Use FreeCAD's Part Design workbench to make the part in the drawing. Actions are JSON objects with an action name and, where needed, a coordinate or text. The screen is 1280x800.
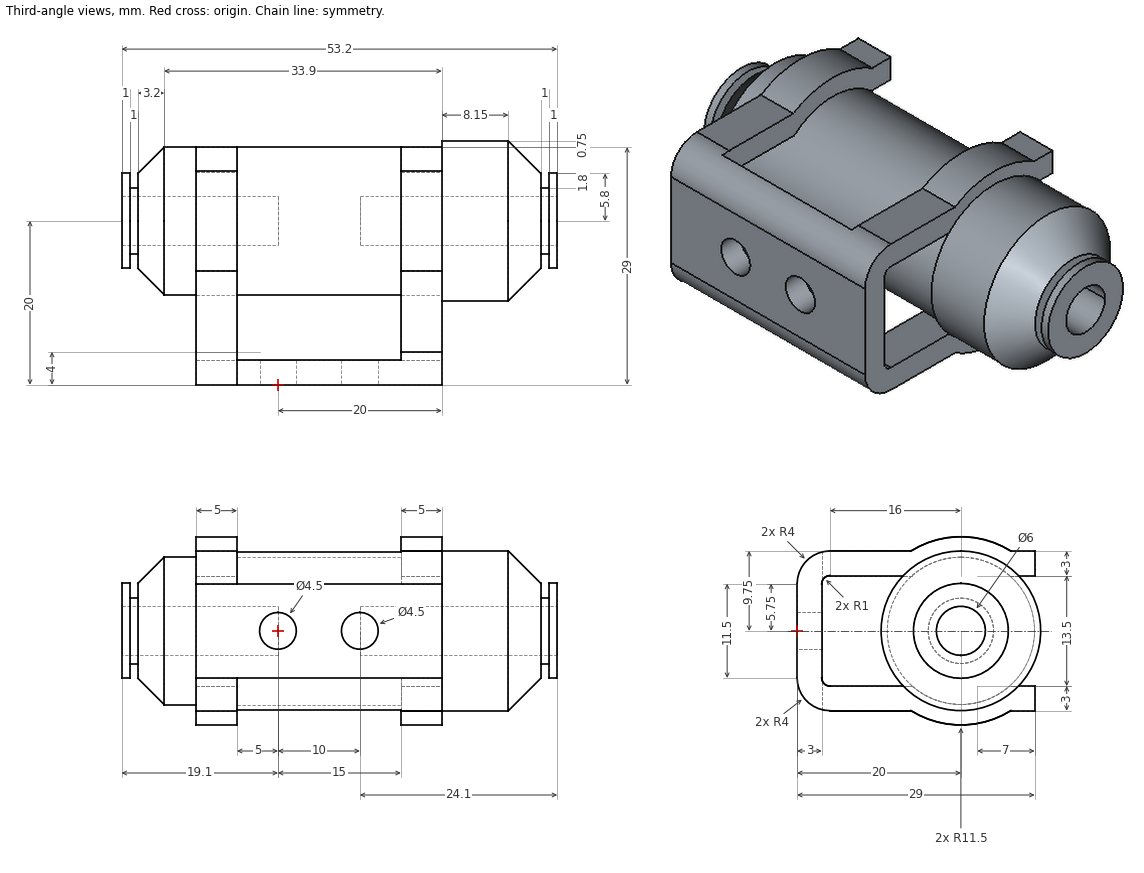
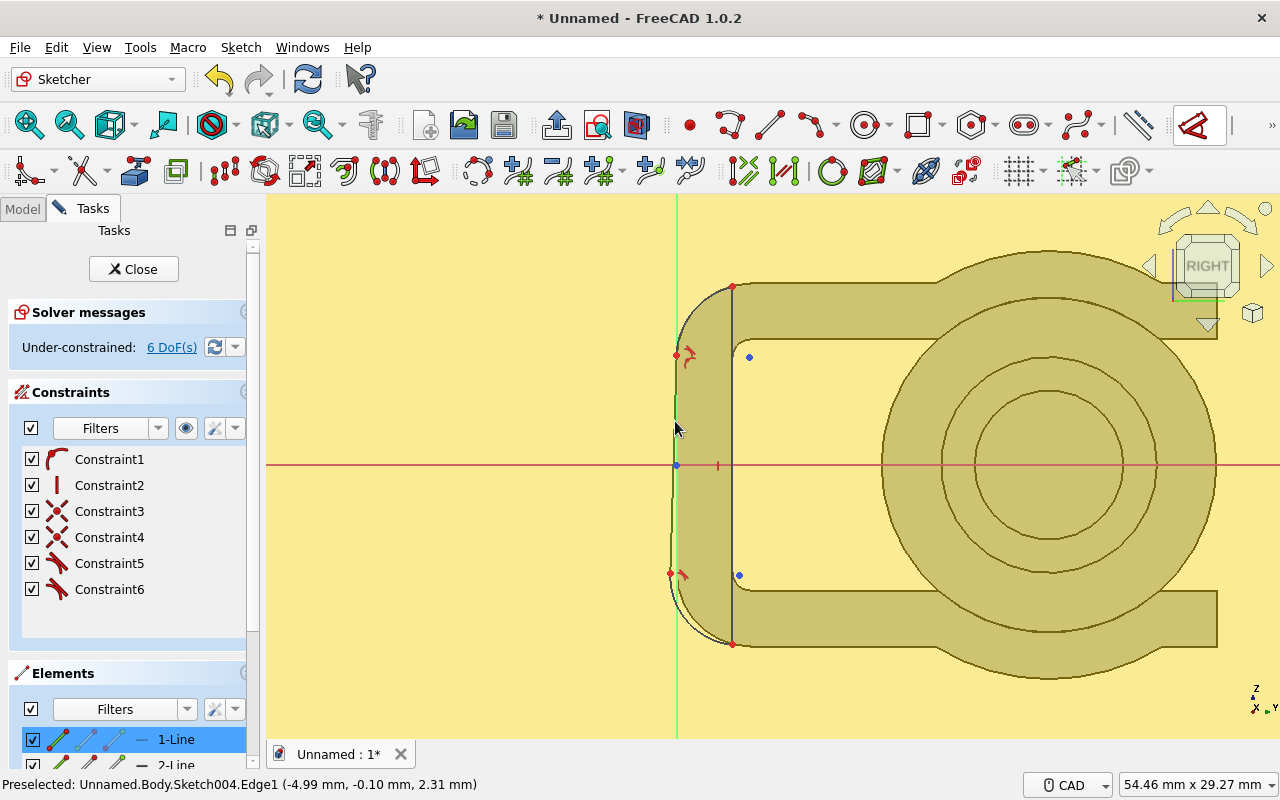
{"action": "key", "text": "v"}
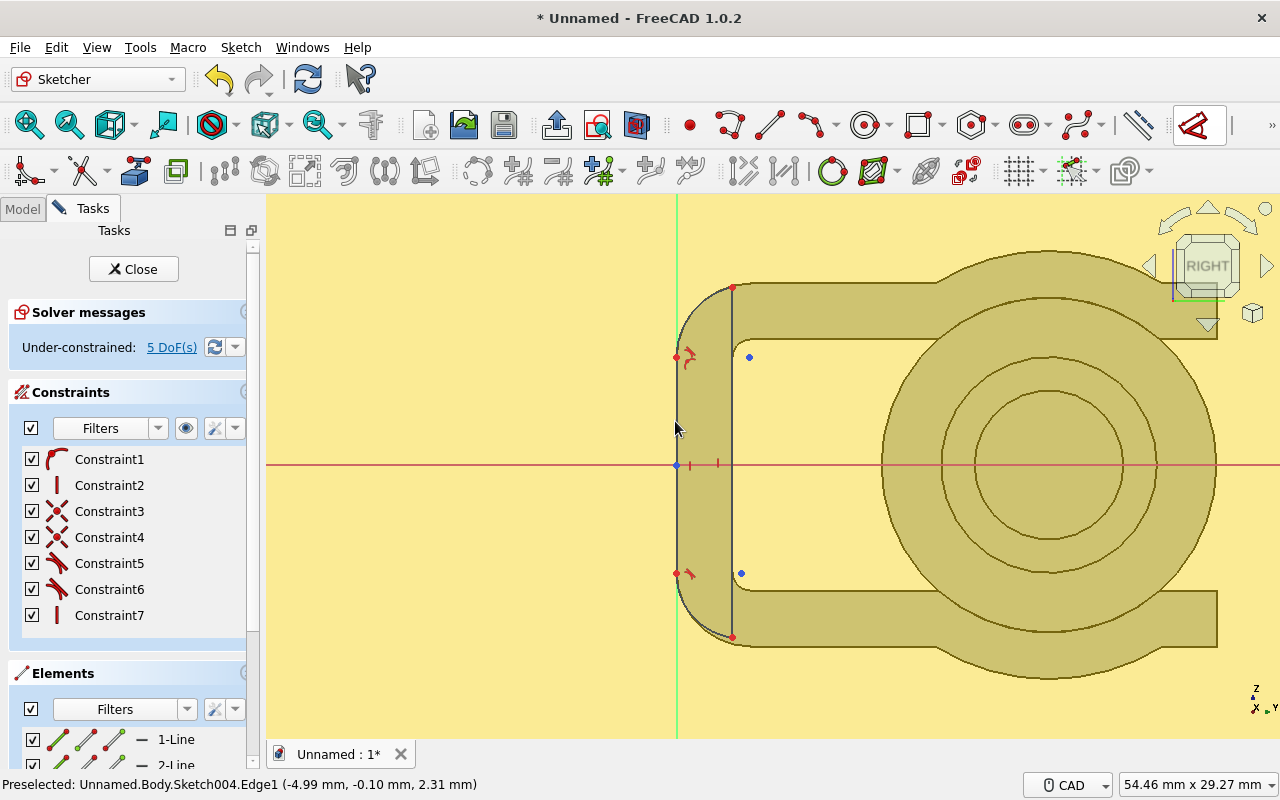
{"action": "left_click", "coordinate": [706, 628]}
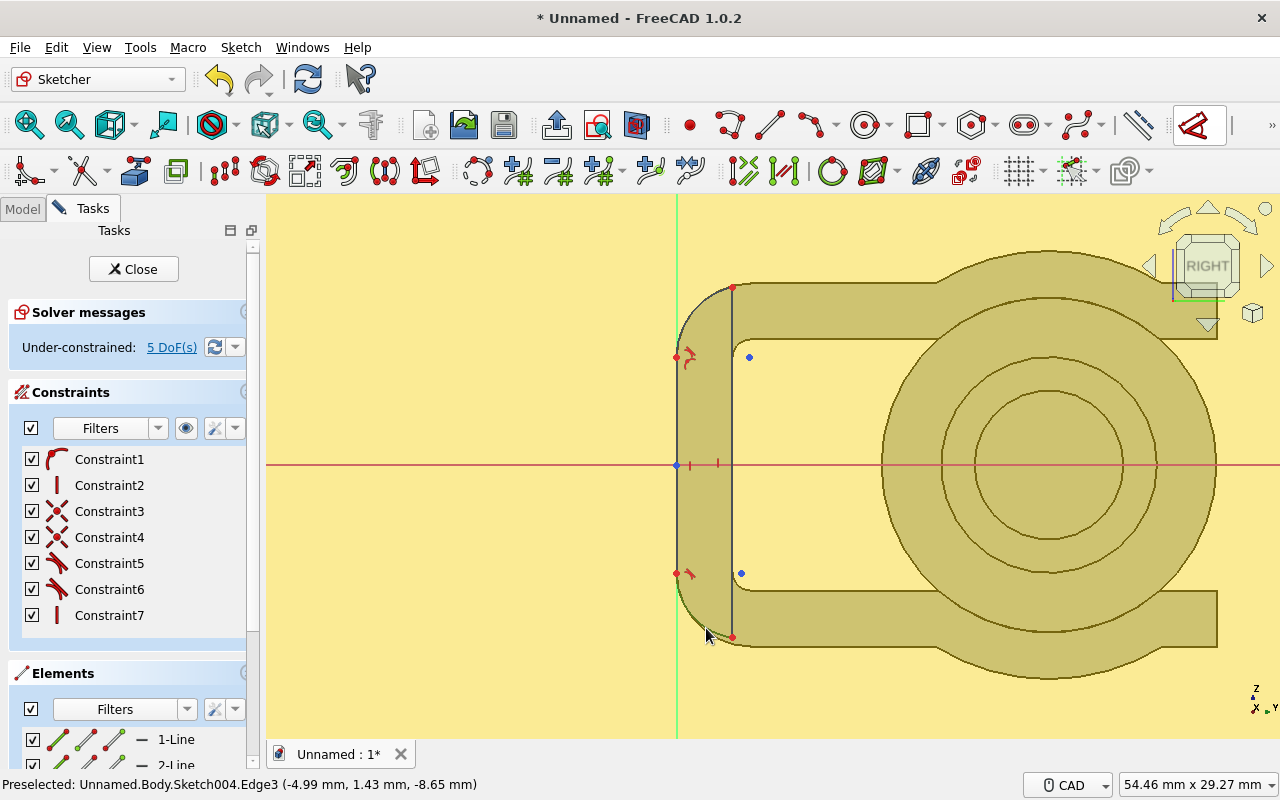
{"action": "left_click", "coordinate": [706, 299]}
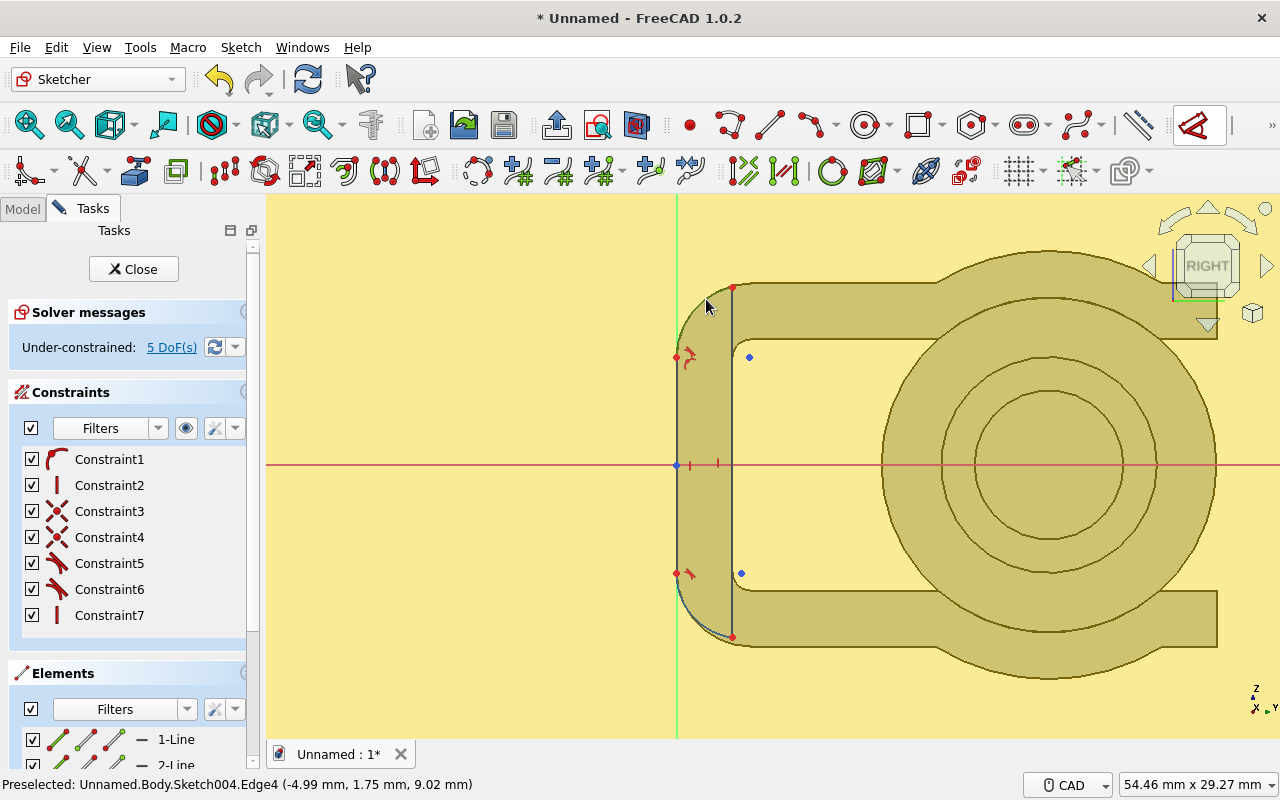
{"action": "key", "text": "e"}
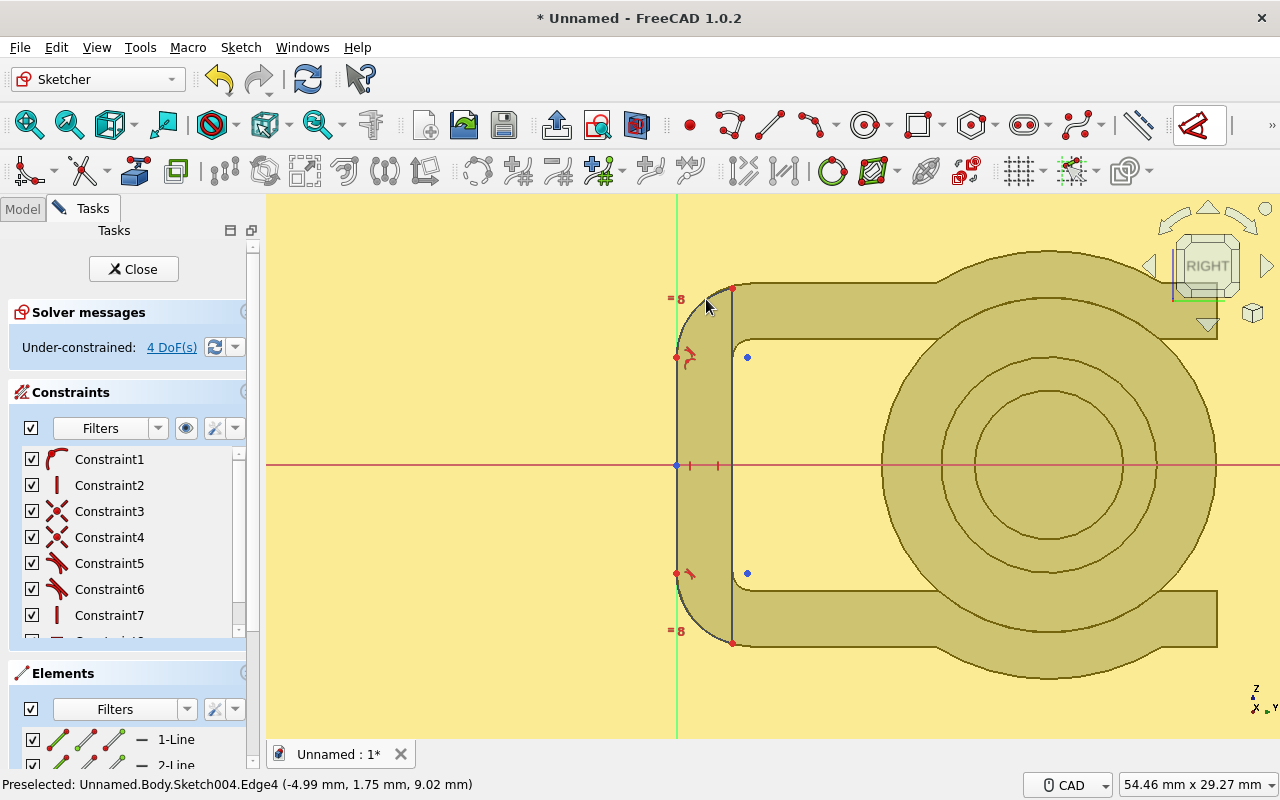
{"action": "left_click", "coordinate": [706, 631]}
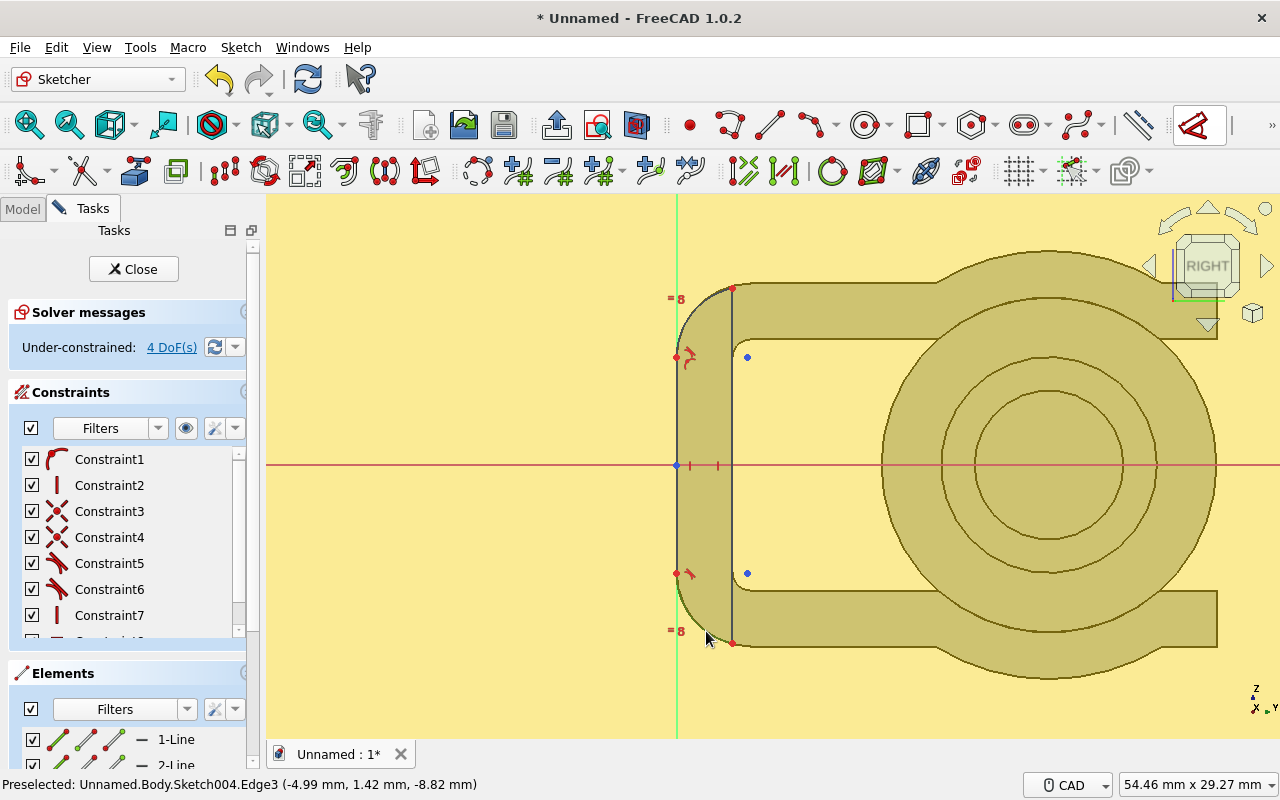
{"action": "key", "text": "k r"}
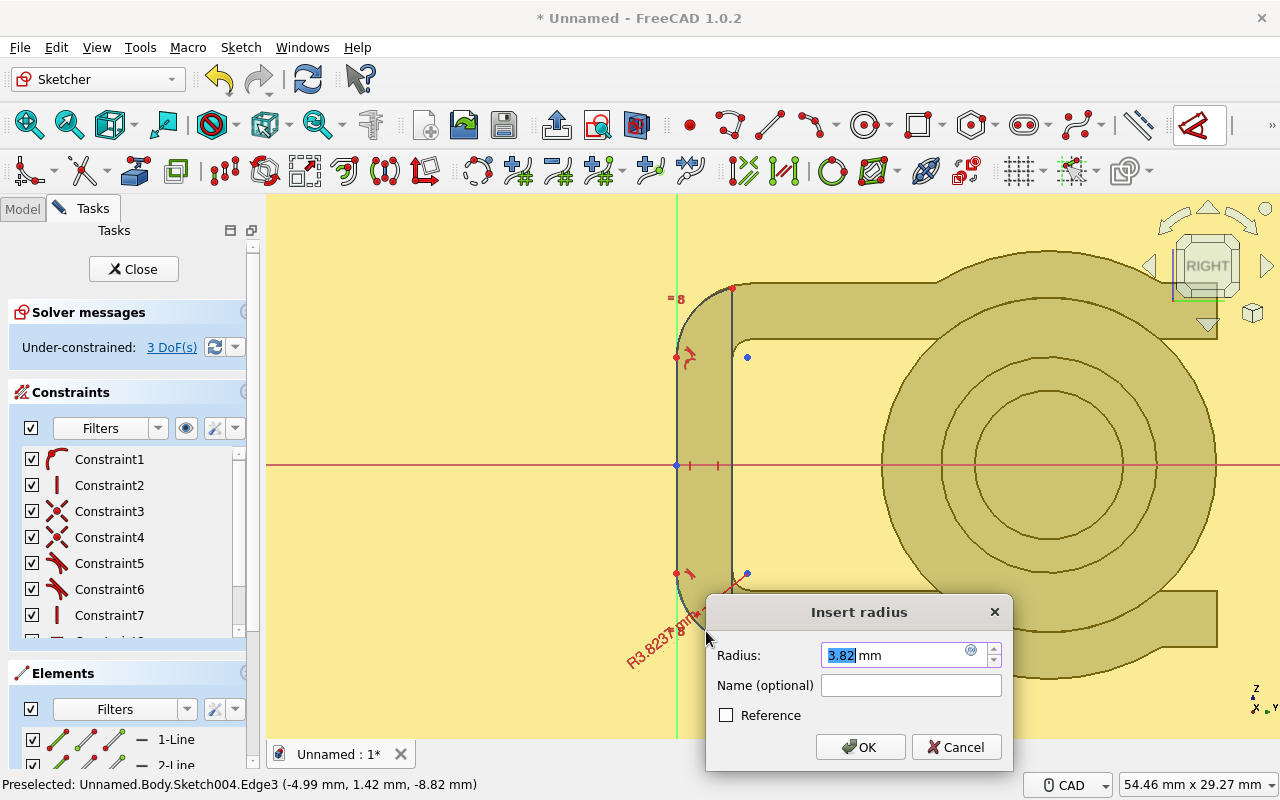
{"action": "type", "text": "4"}
{"action": "key", "text": "Return"}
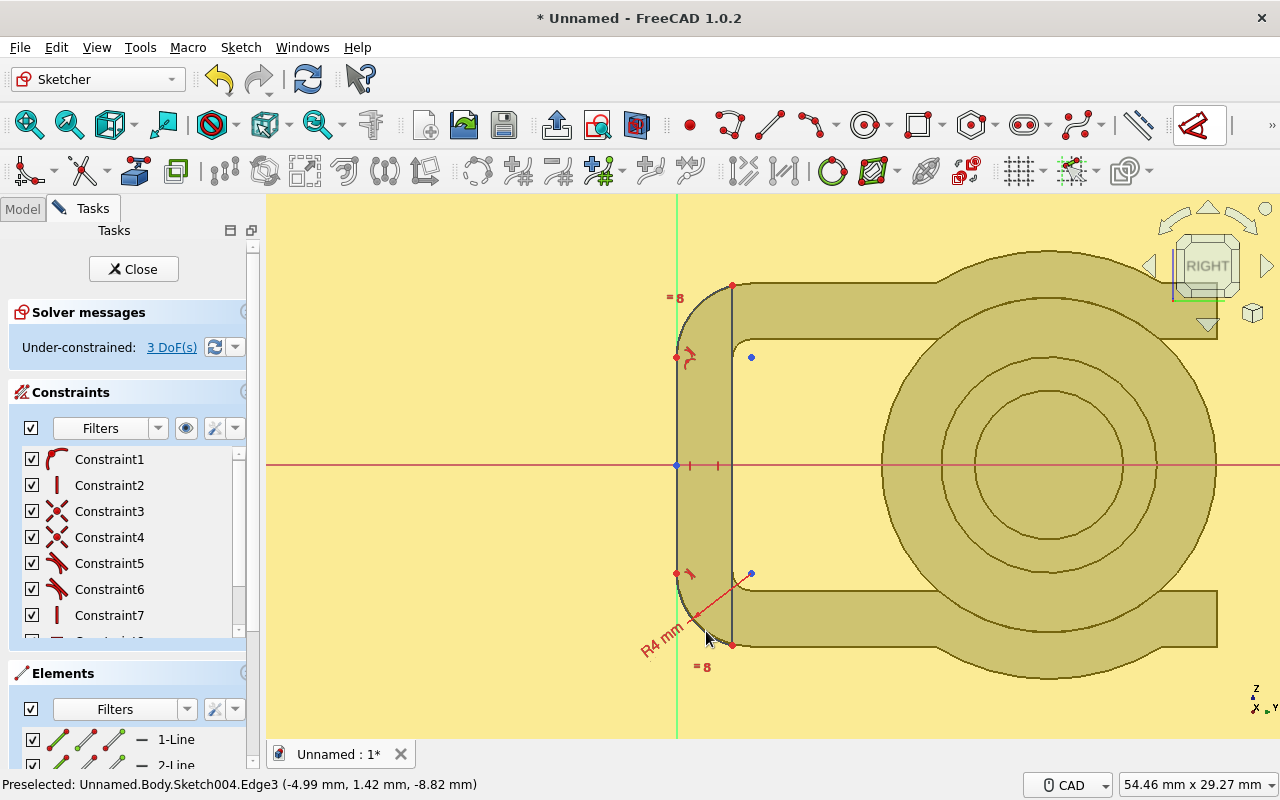
{"action": "left_click", "coordinate": [732, 646]}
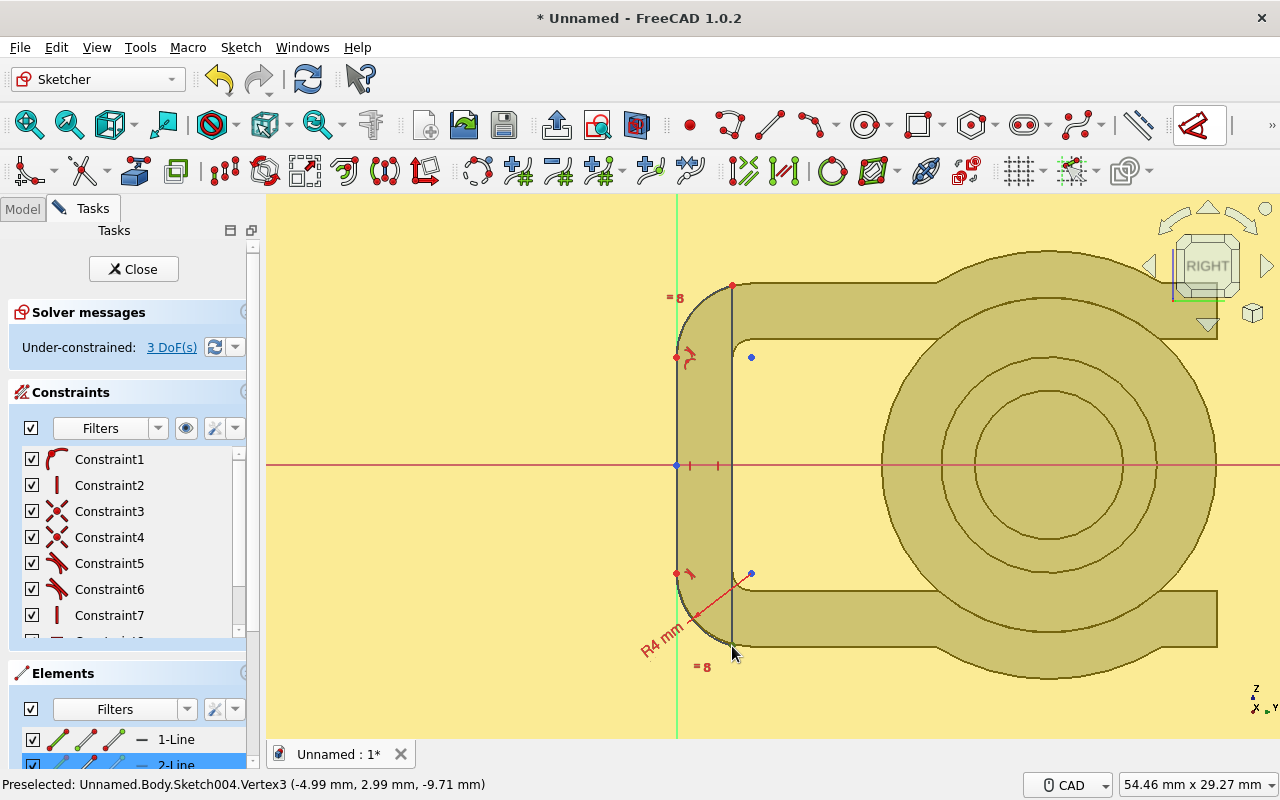
{"action": "key", "text": "l"}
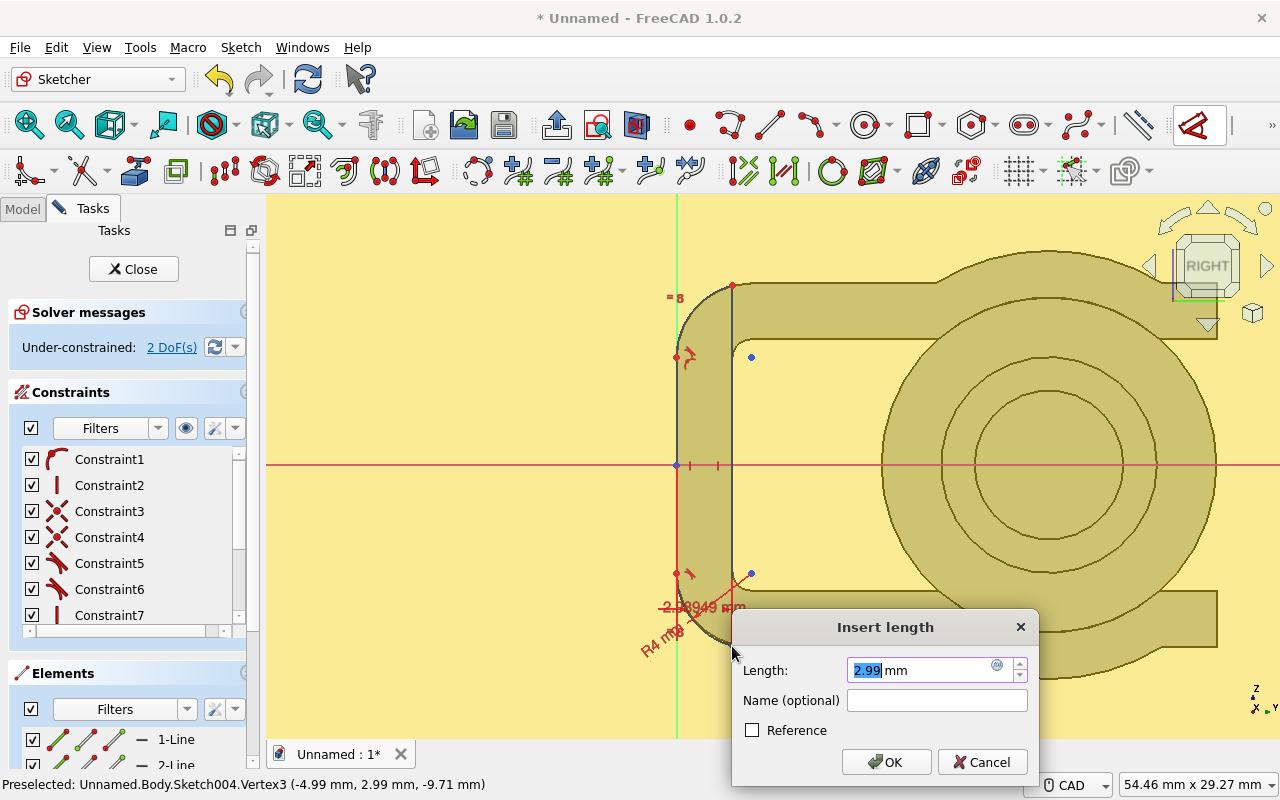
{"action": "type", "text": "3"}
{"action": "key", "text": "Return"}